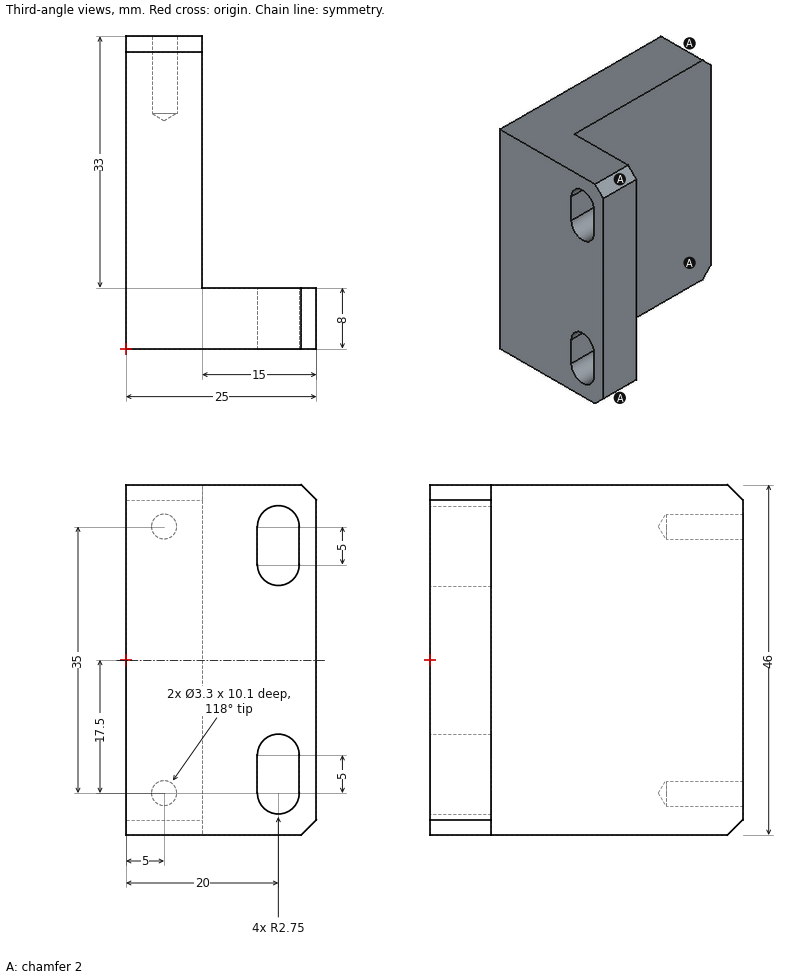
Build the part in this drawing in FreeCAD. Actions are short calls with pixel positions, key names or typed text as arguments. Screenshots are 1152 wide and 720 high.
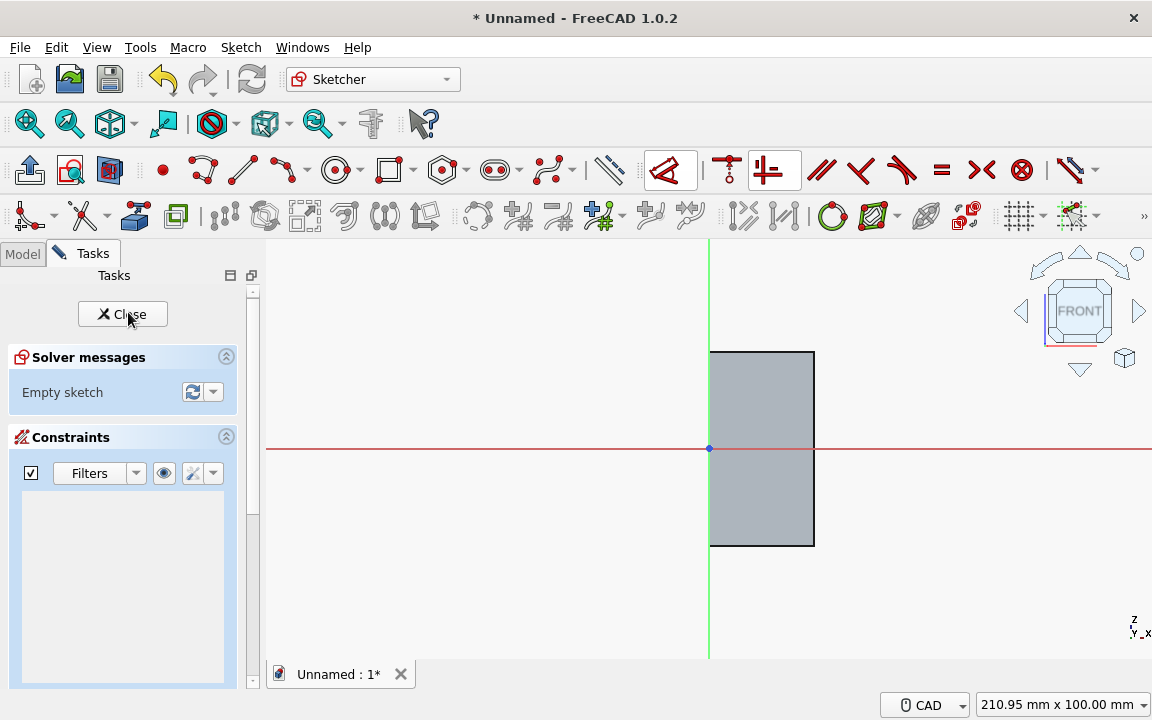
scroll(987, 449, up, 2)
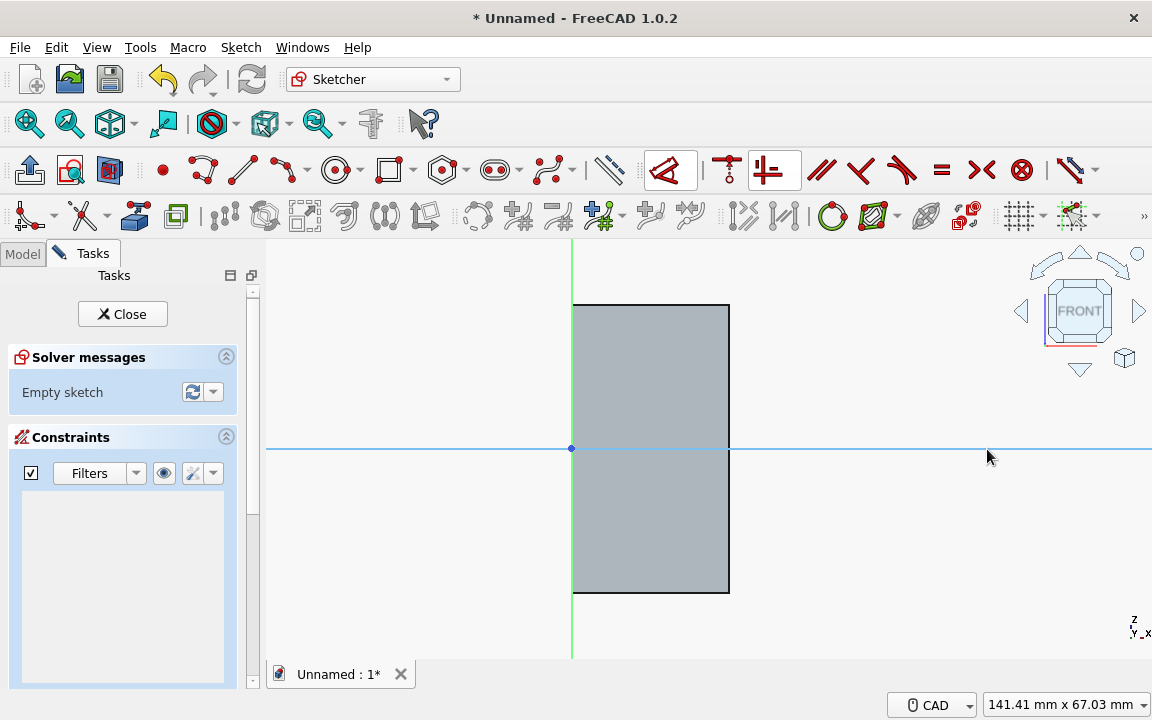
click(496, 170)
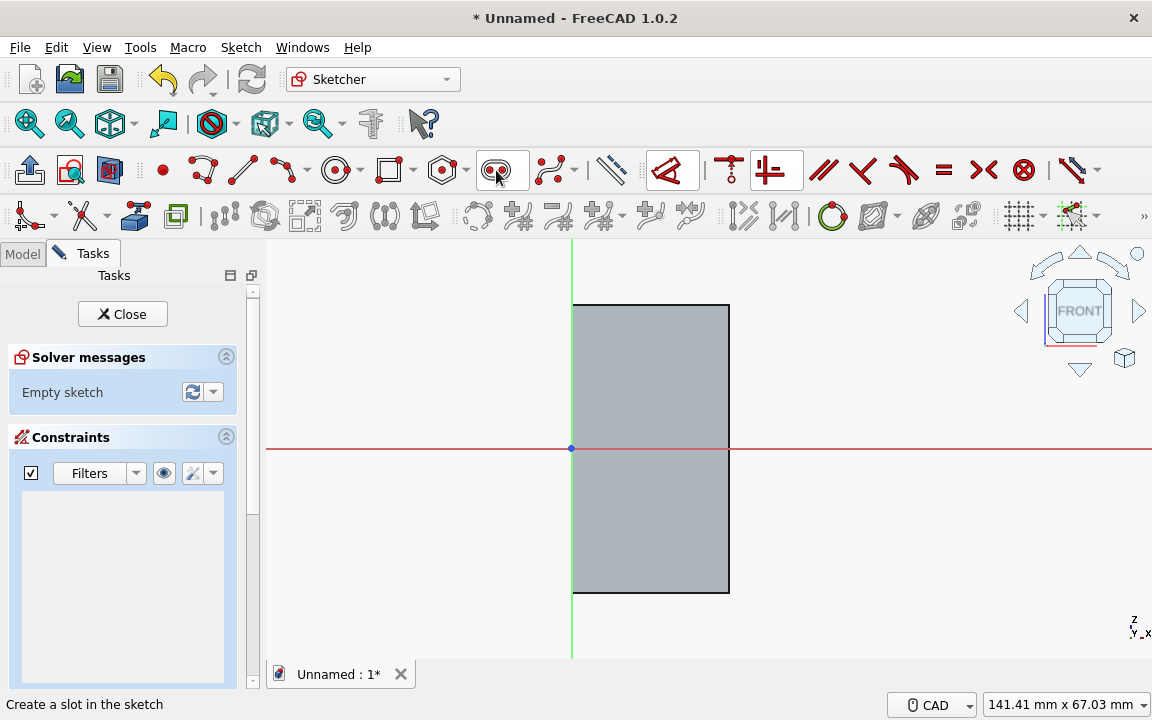
scroll(697, 558, up, 2)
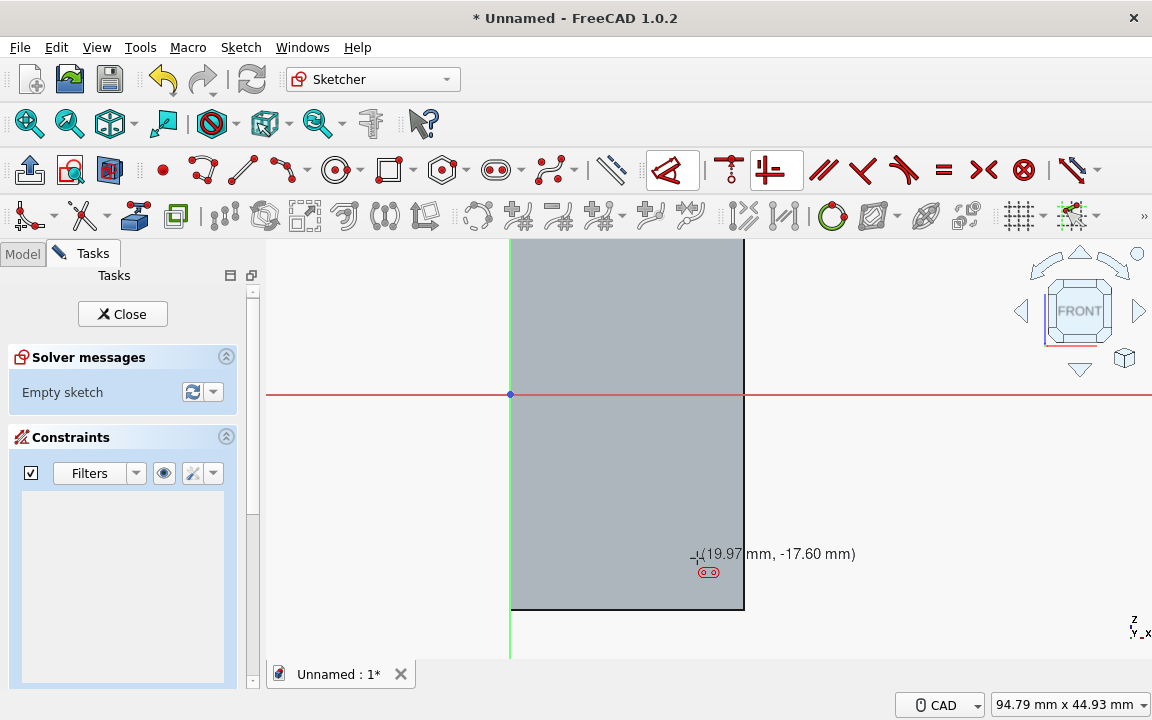
click(697, 558)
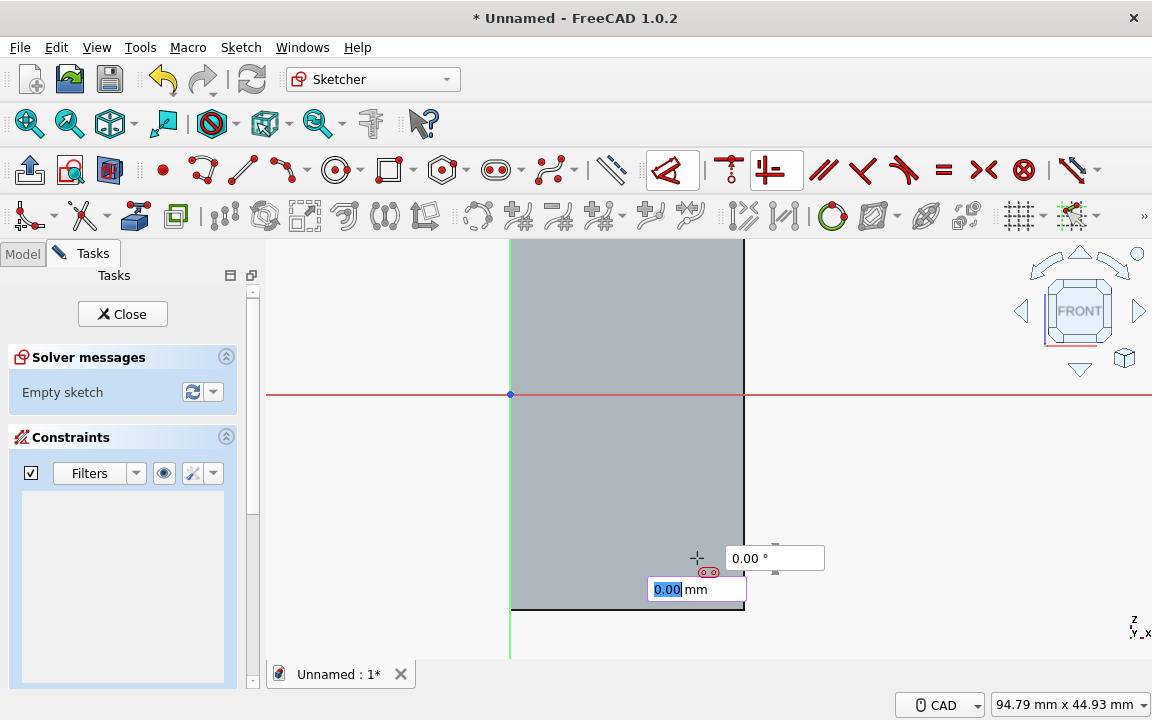
click(697, 511)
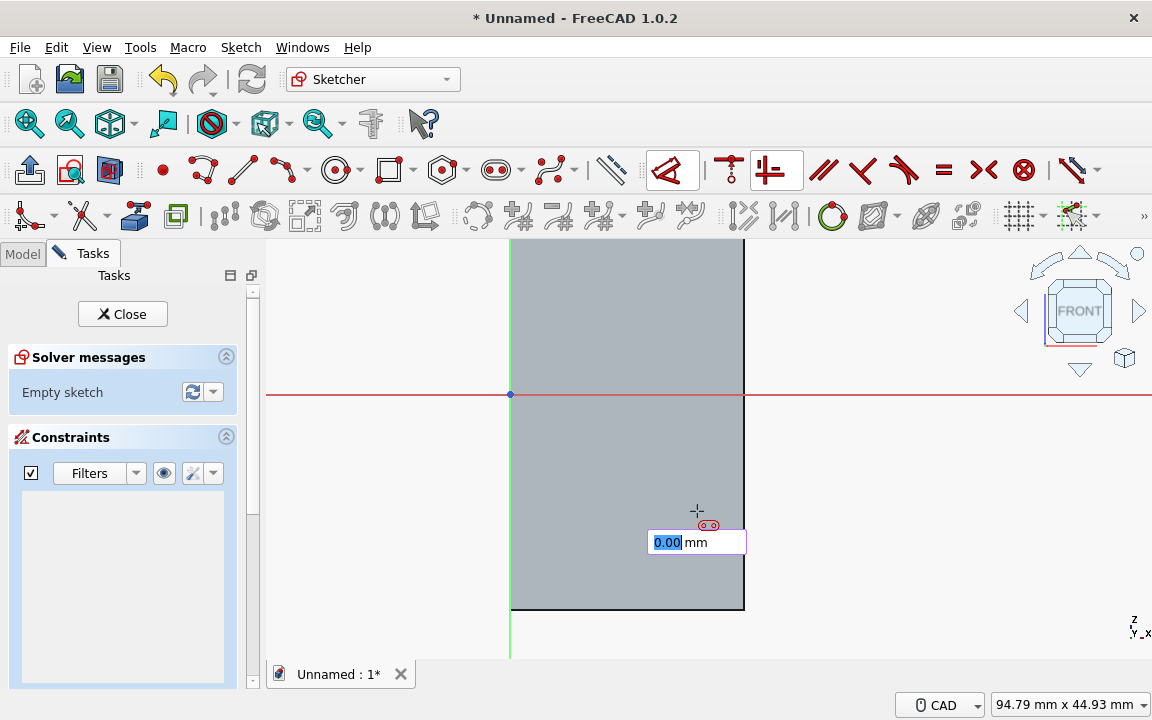
click(723, 535)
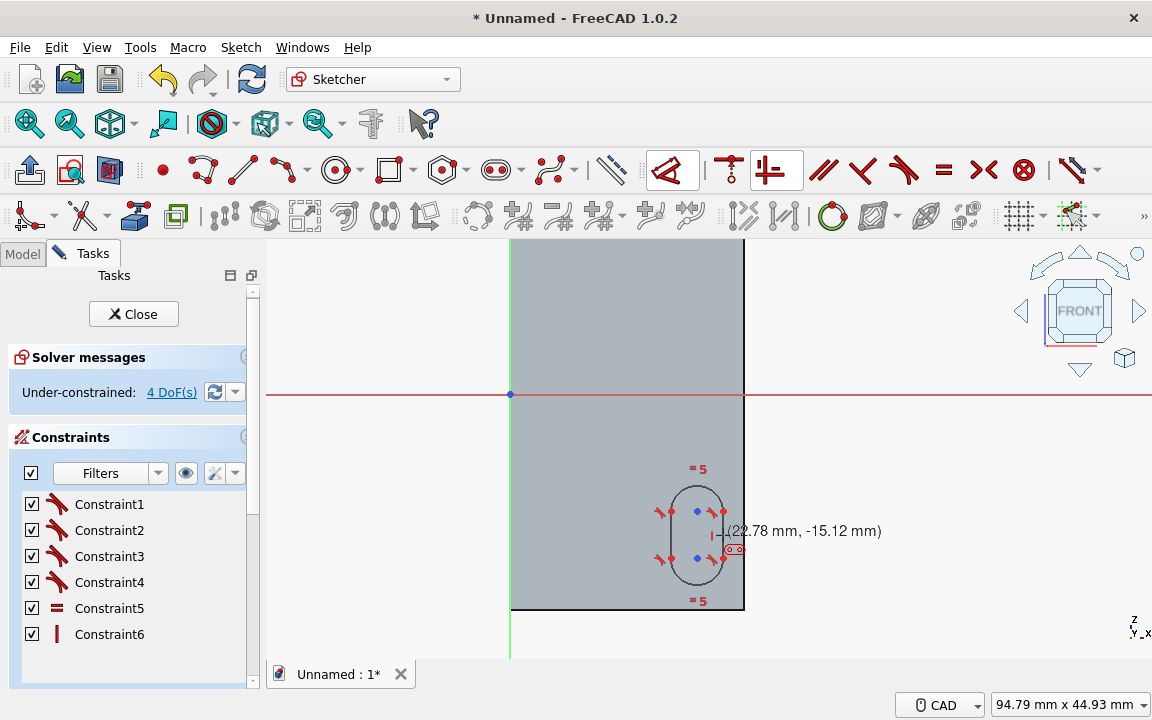
click(697, 278)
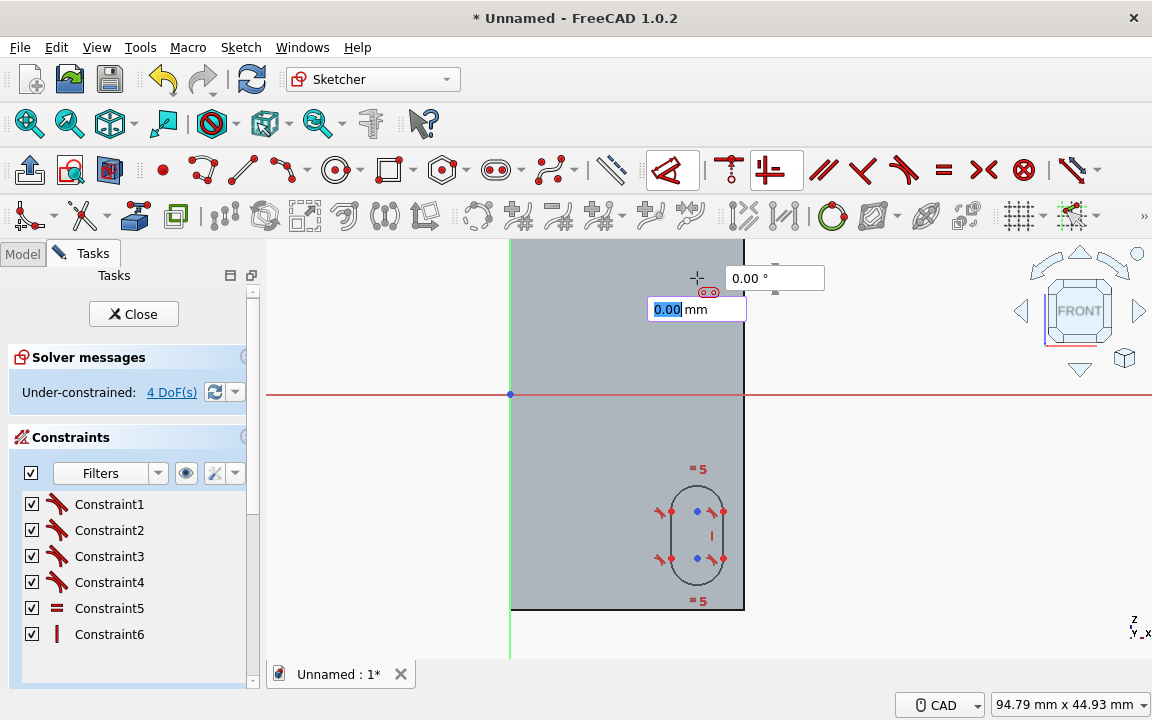
scroll(689, 560, down, 2)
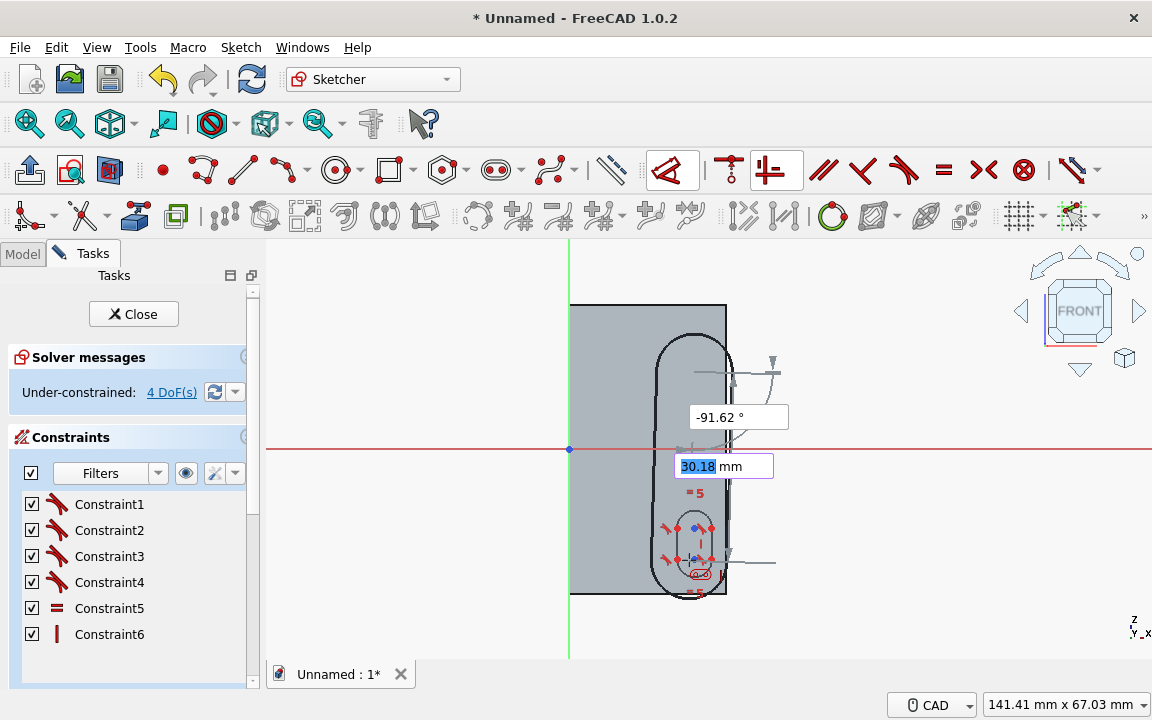
click(695, 340)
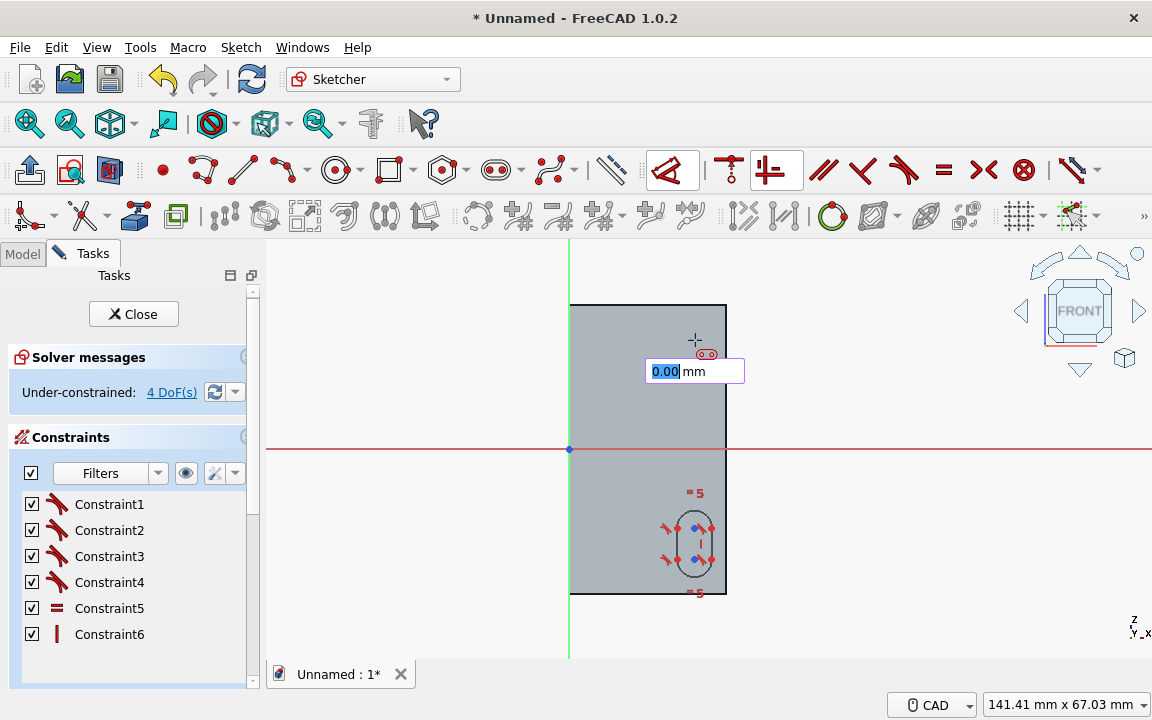
click(712, 355)
key(Escape)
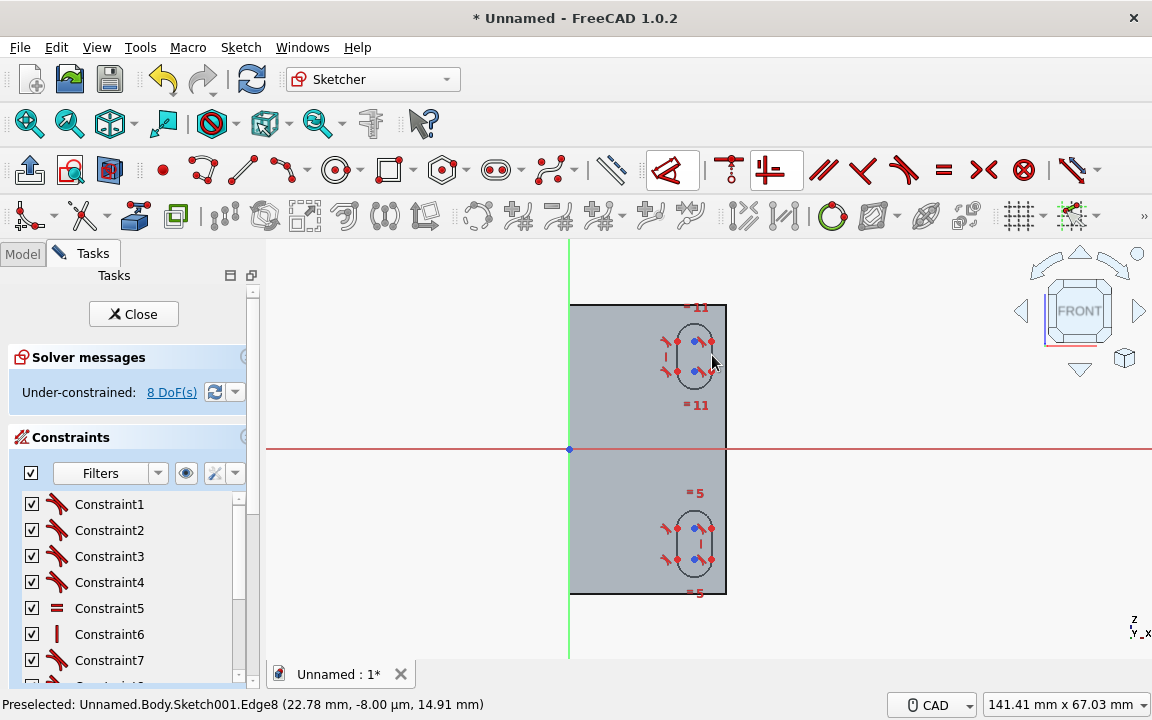
click(684, 574)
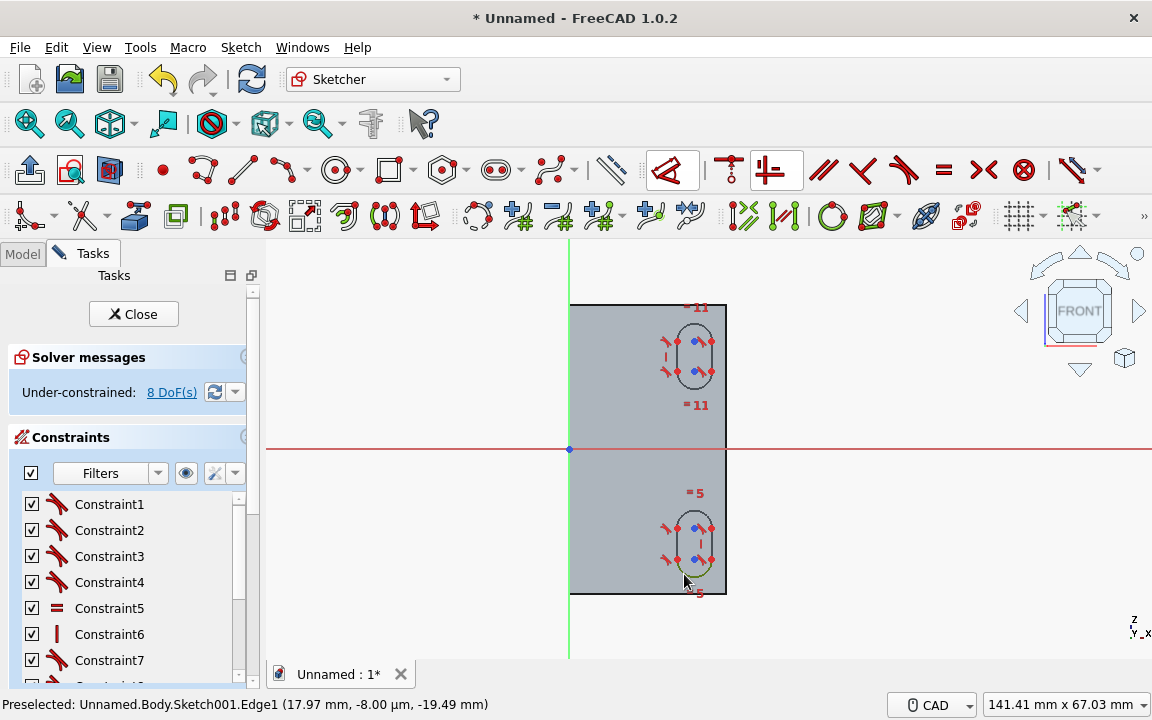
click(684, 386)